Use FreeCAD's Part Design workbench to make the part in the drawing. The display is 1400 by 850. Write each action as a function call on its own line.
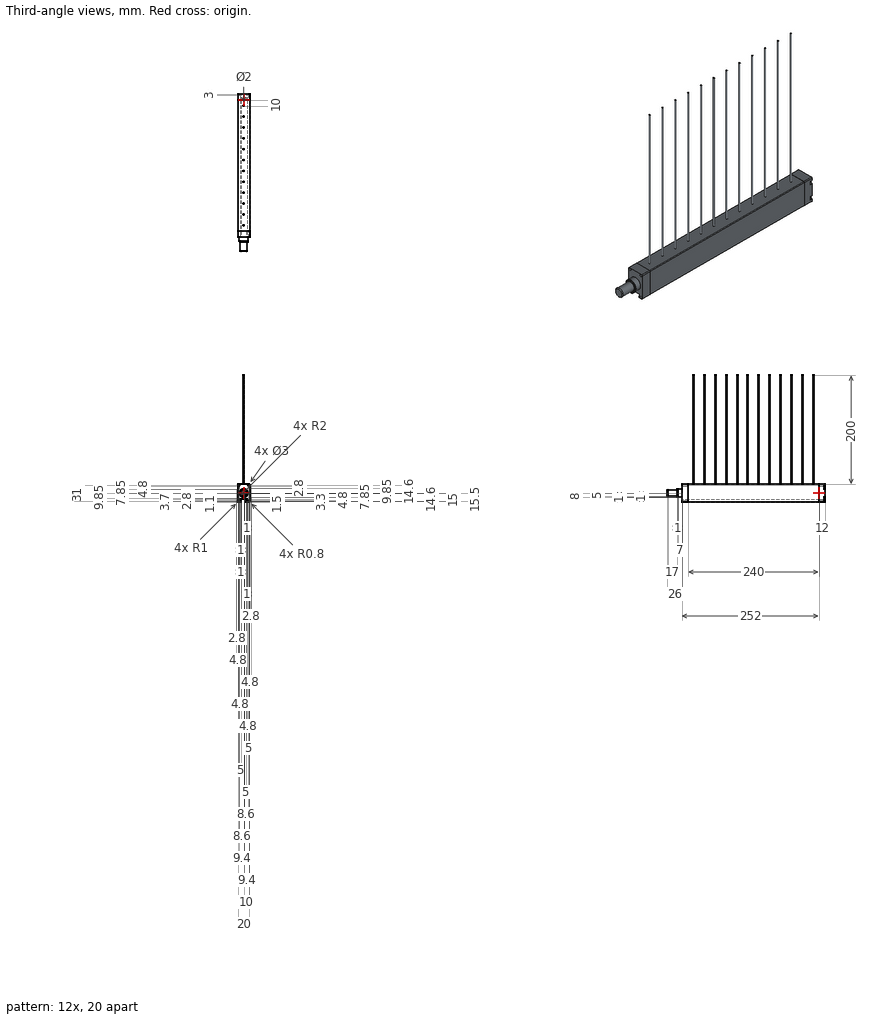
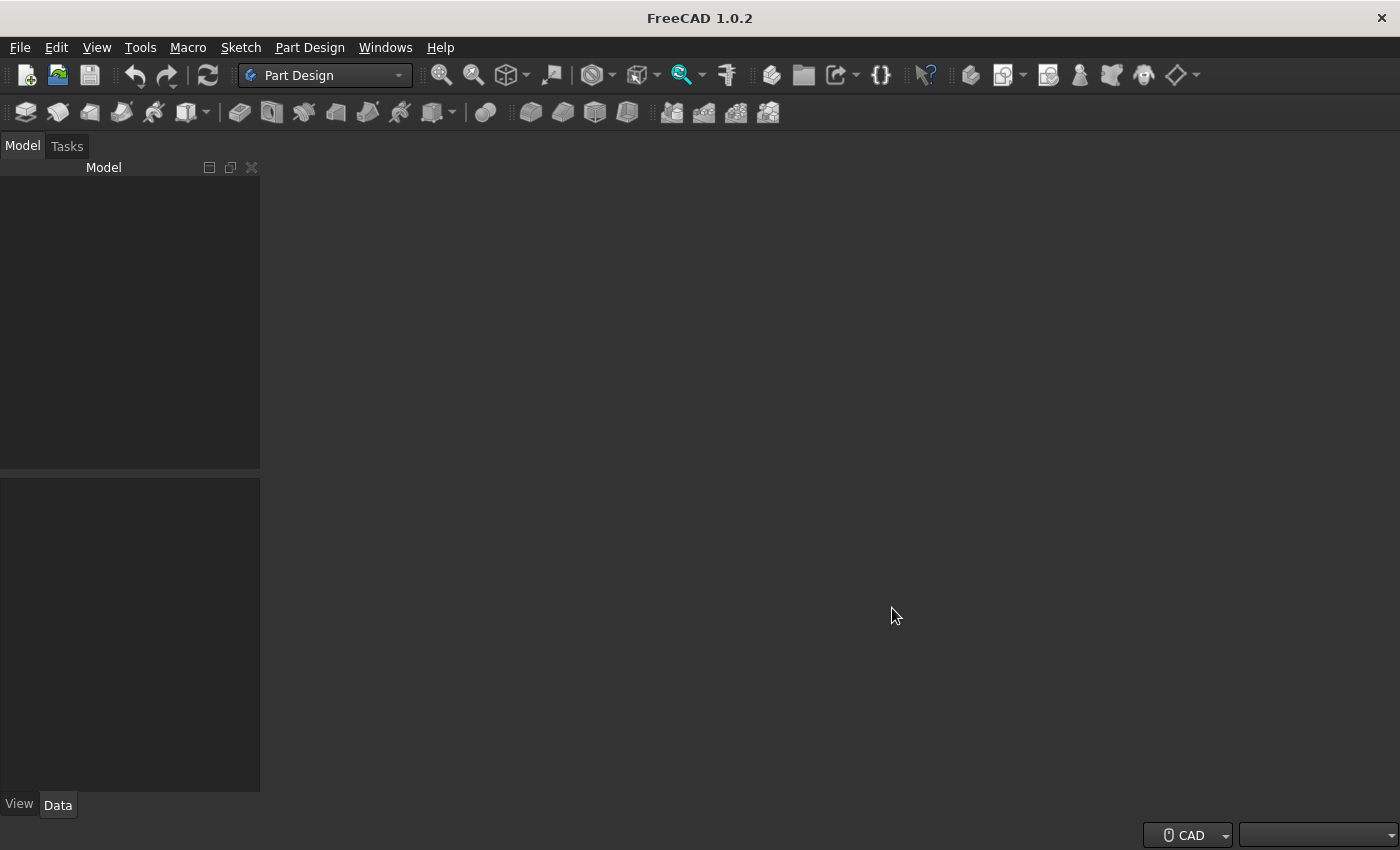
click(26, 76)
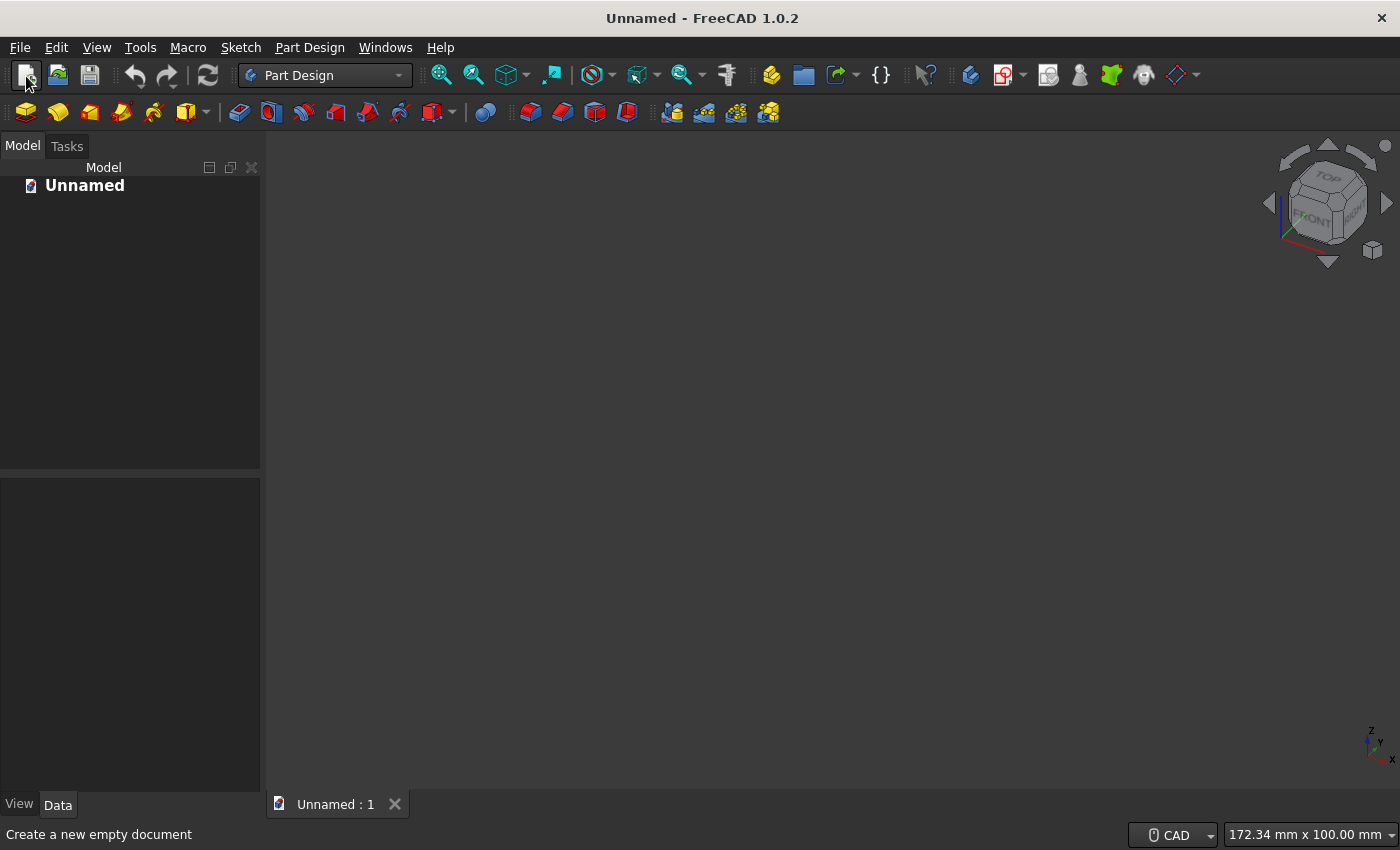
click(1004, 76)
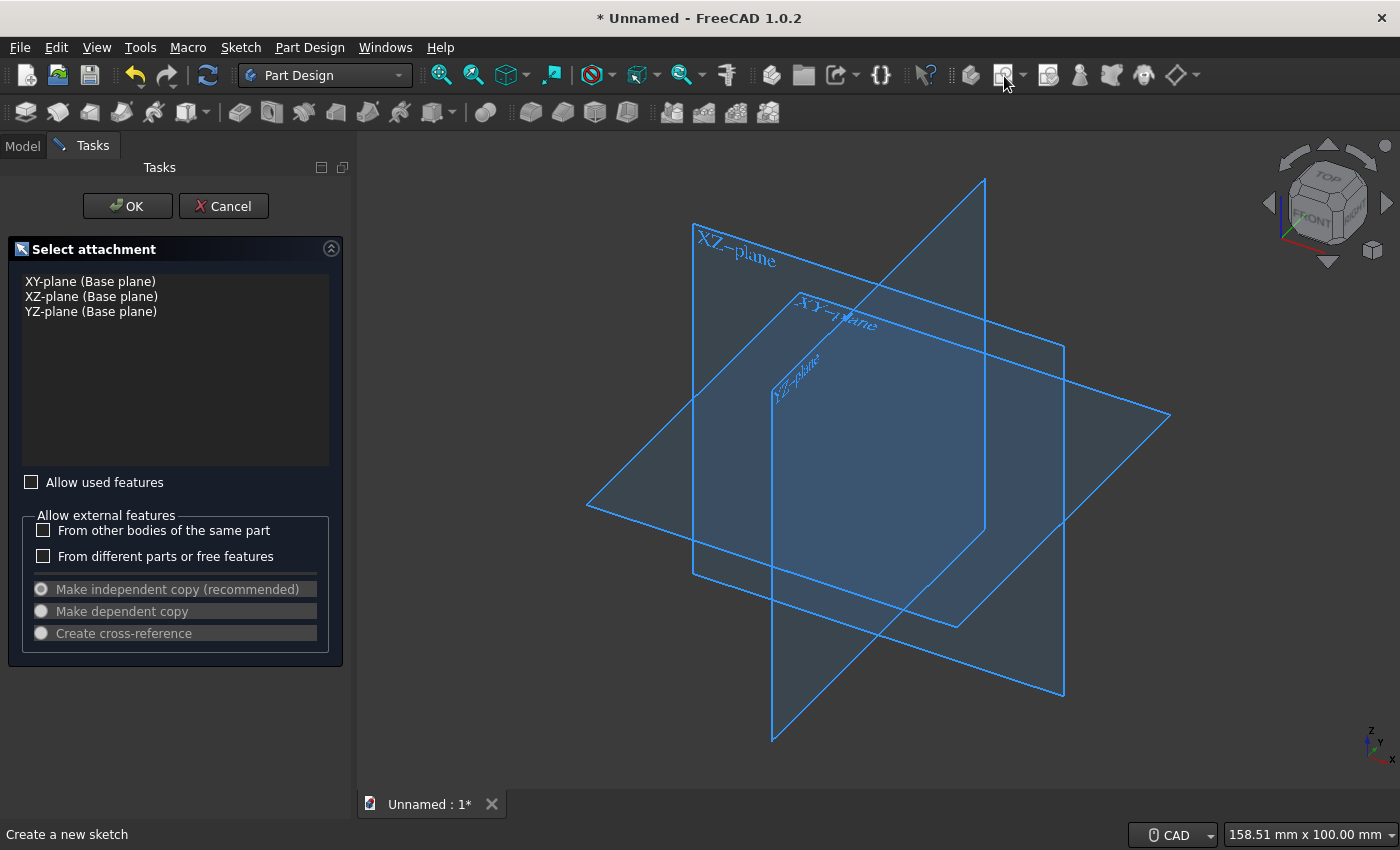
click(82, 296)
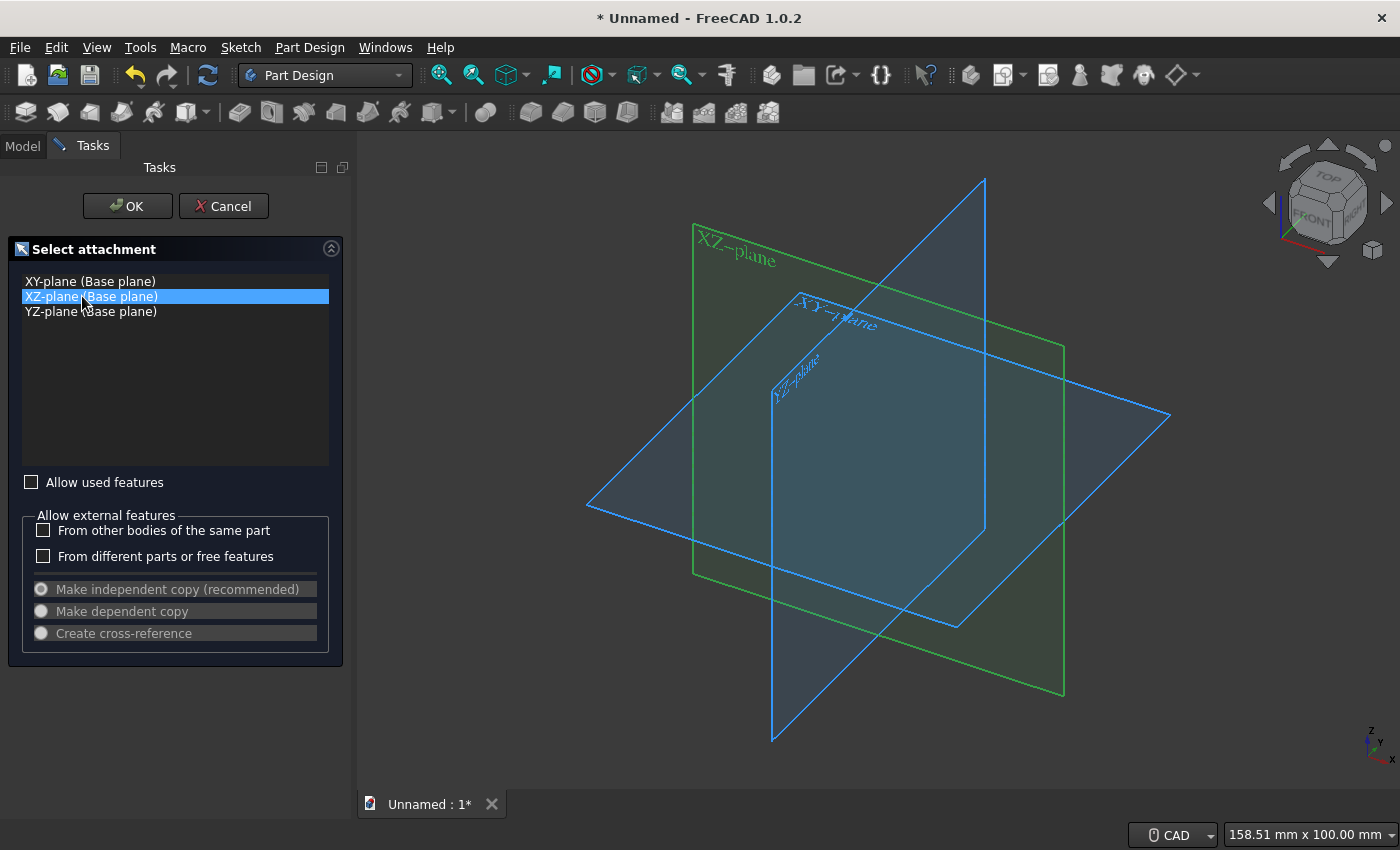
click(128, 206)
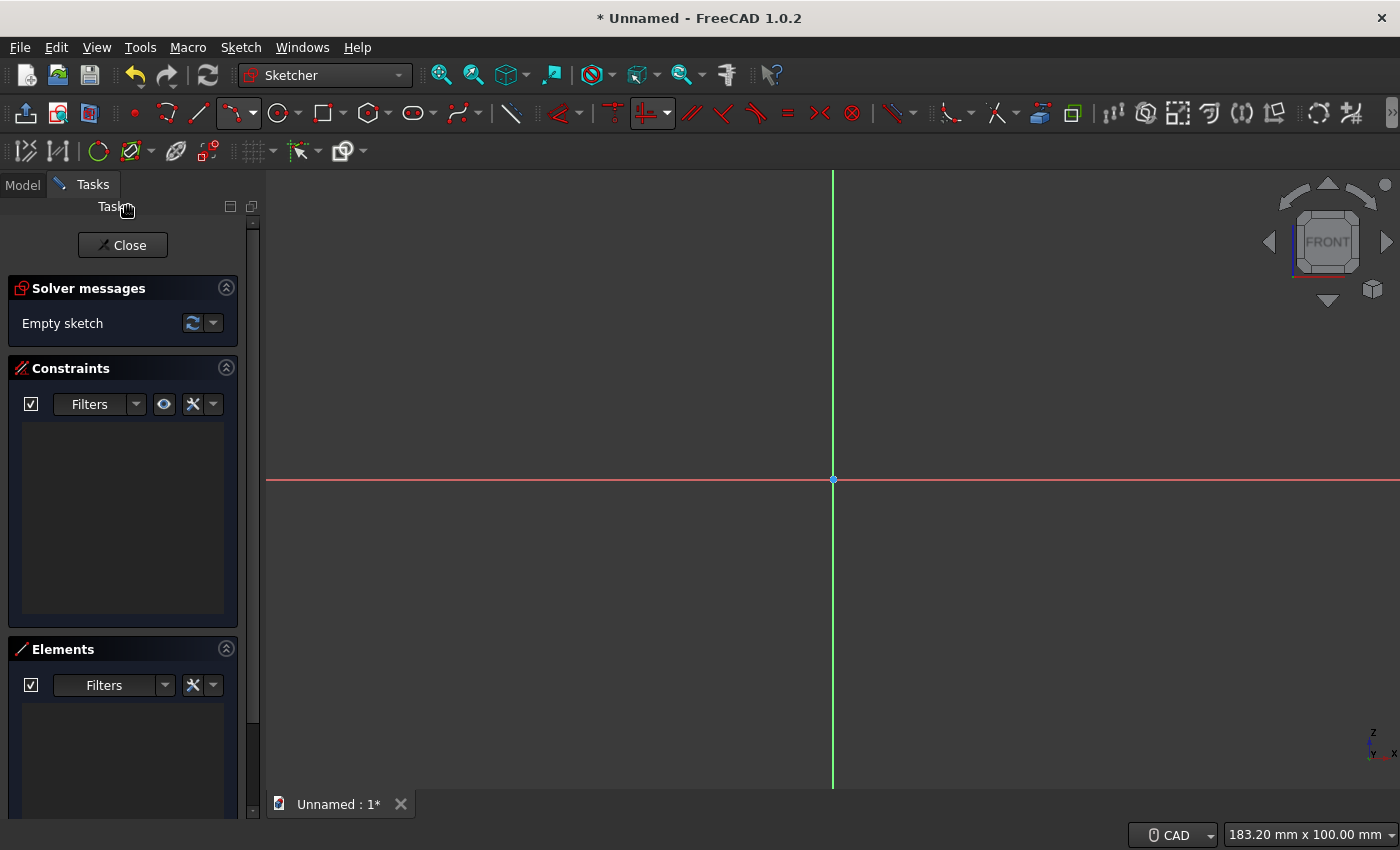
scroll(916, 480, up, 3)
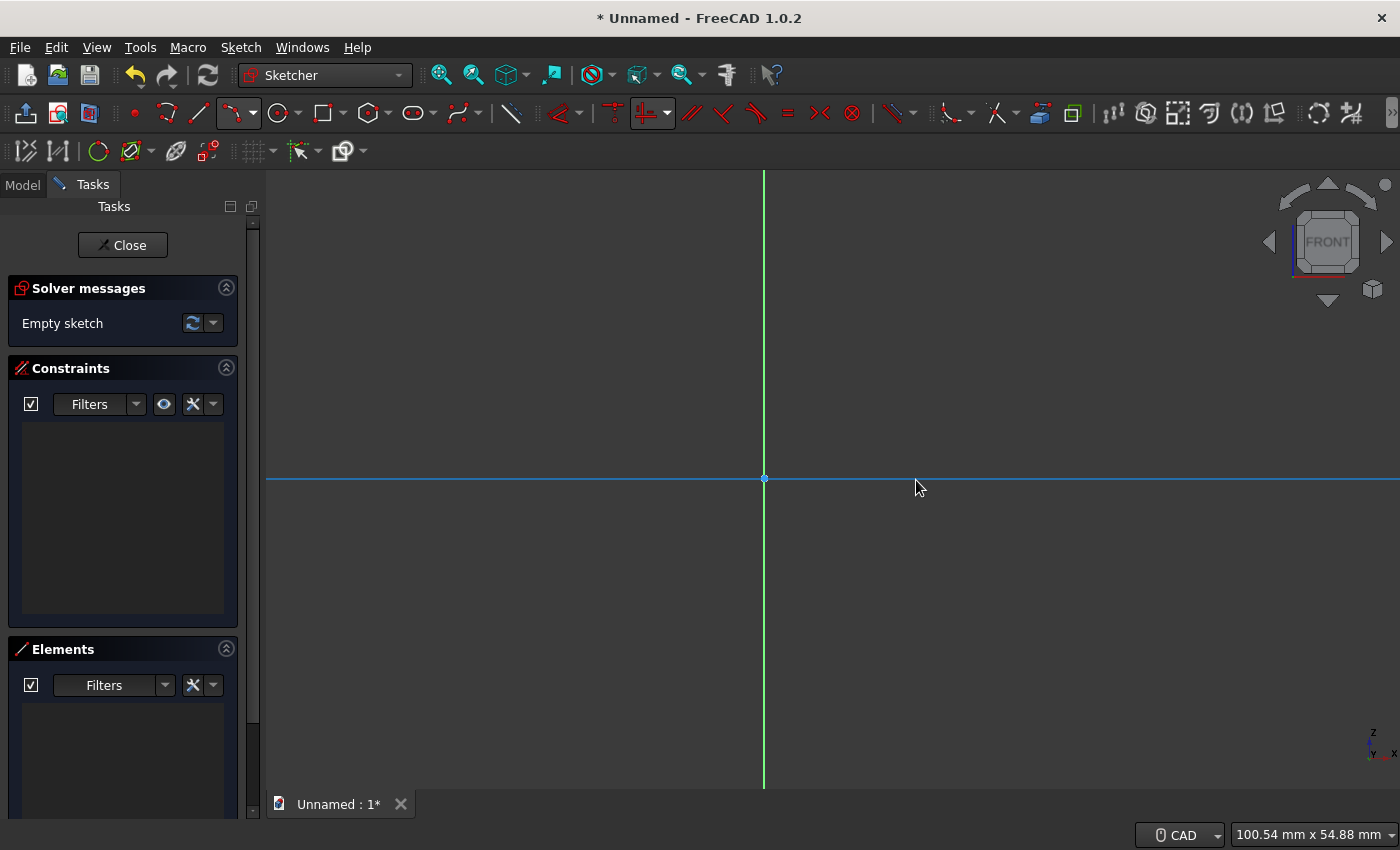
click(200, 114)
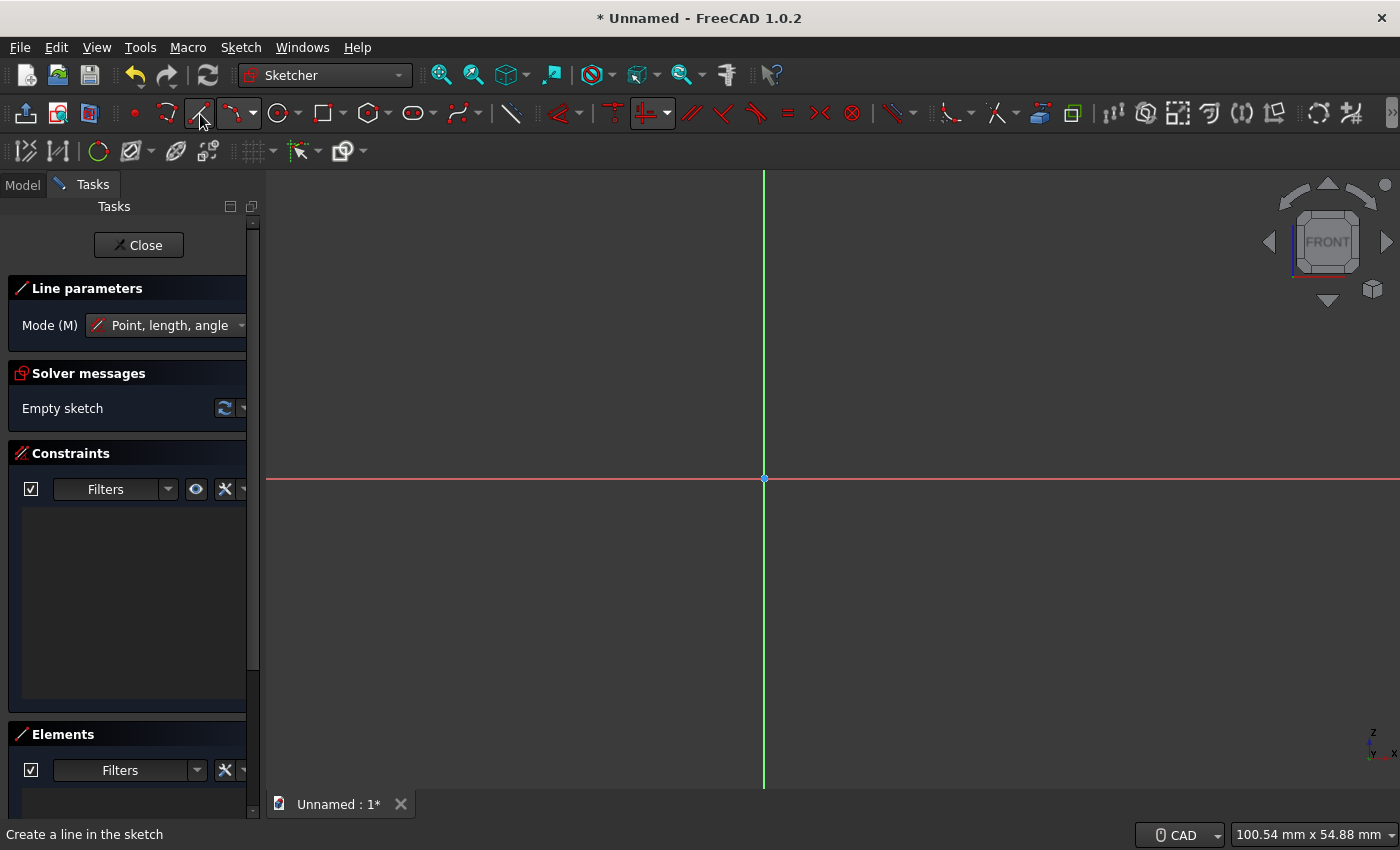
click(640, 653)
click(640, 304)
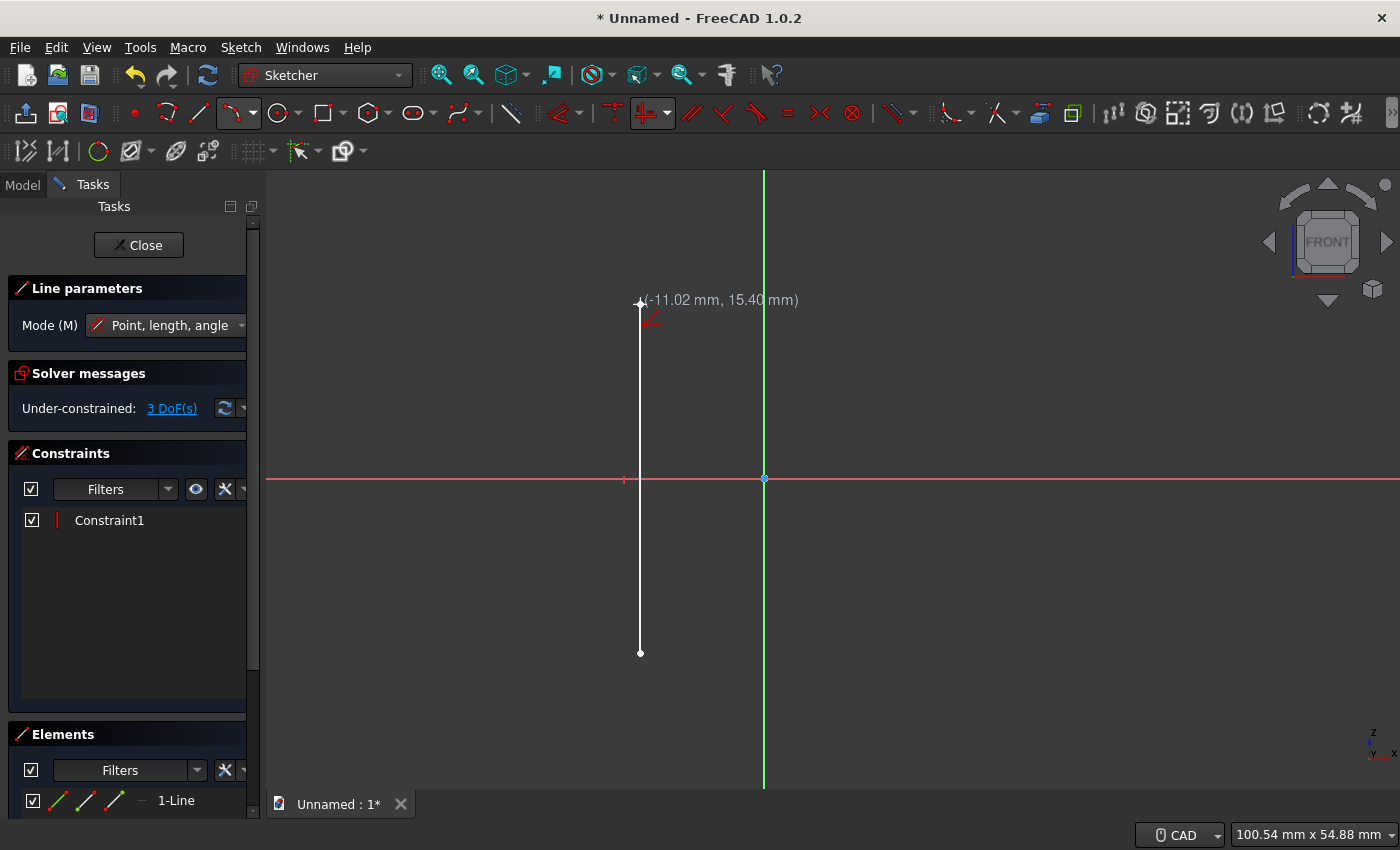
click(652, 293)
click(877, 293)